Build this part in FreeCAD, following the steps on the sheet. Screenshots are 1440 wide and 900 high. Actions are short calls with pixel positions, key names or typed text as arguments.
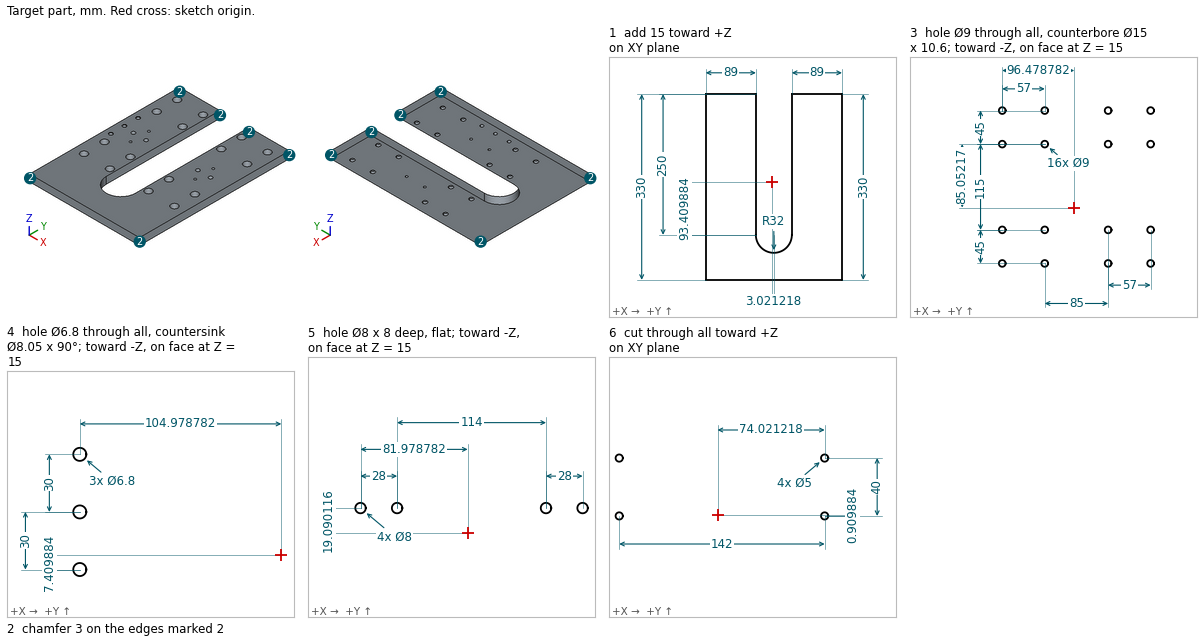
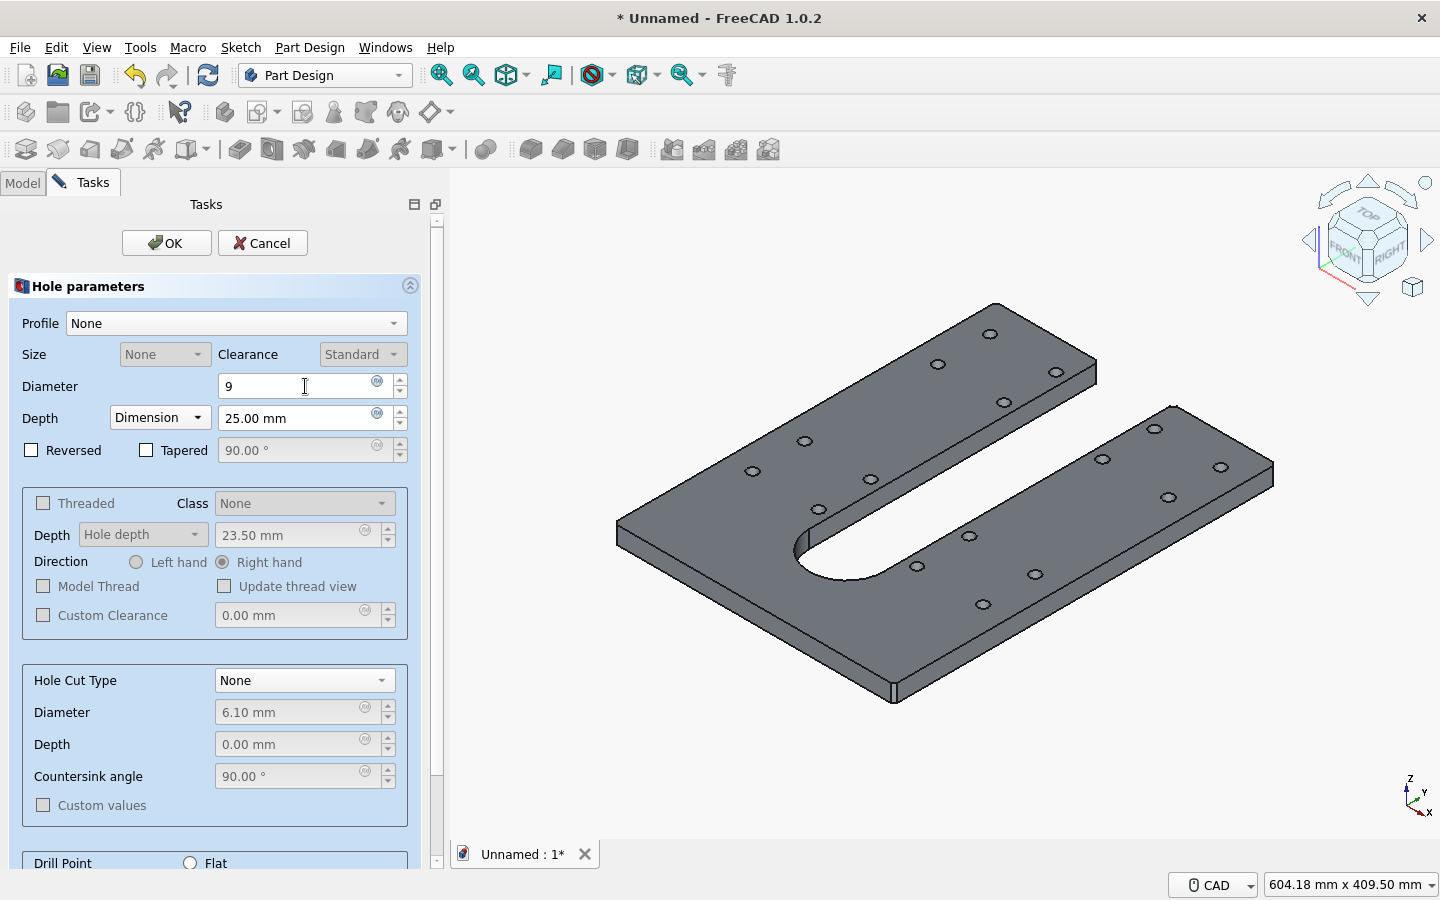
click(161, 418)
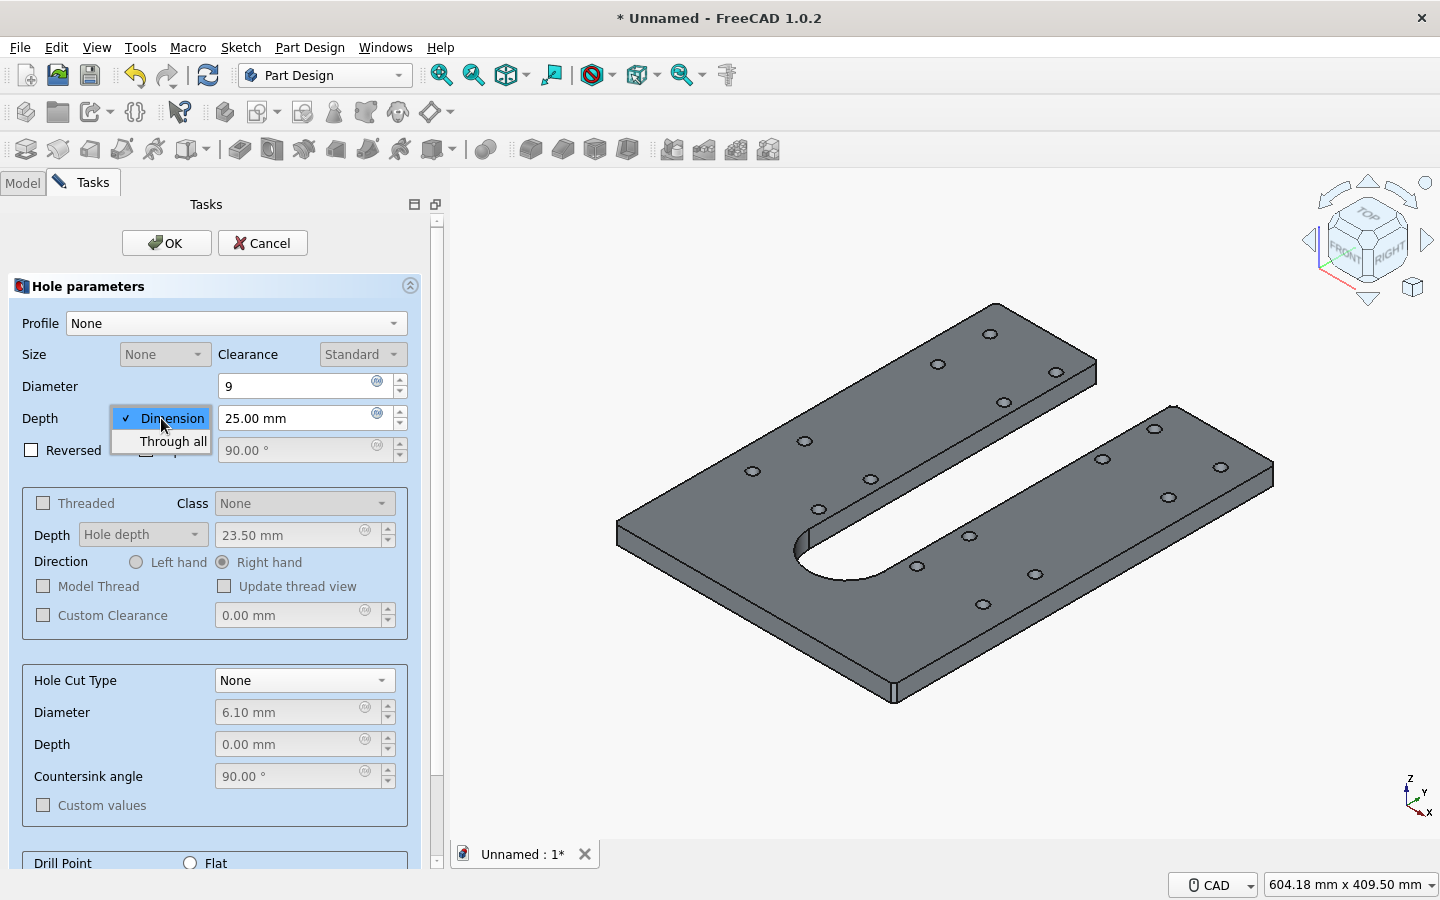
click(160, 442)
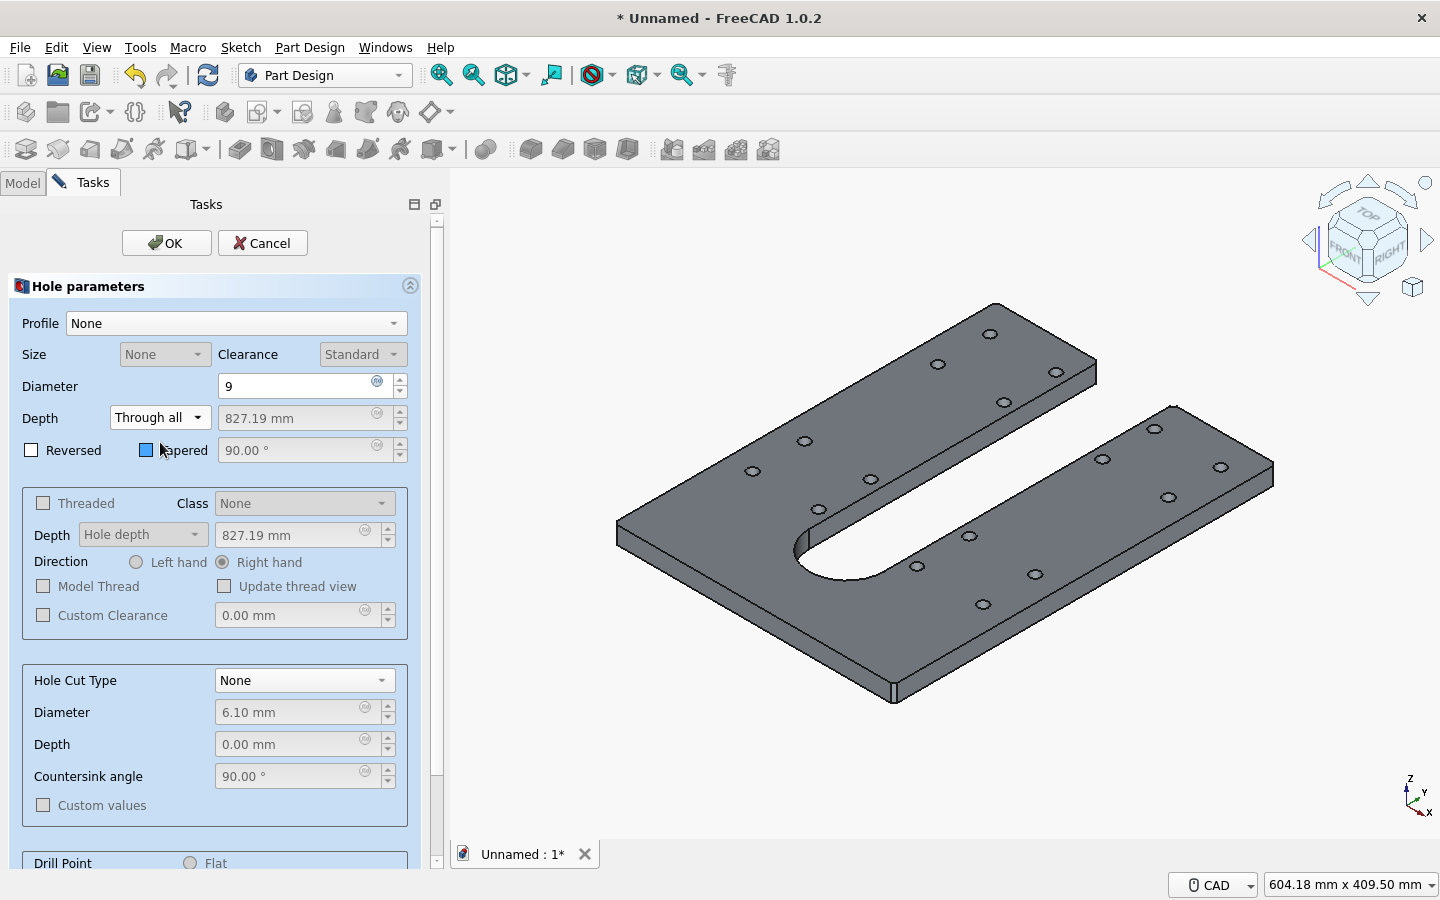
click(306, 680)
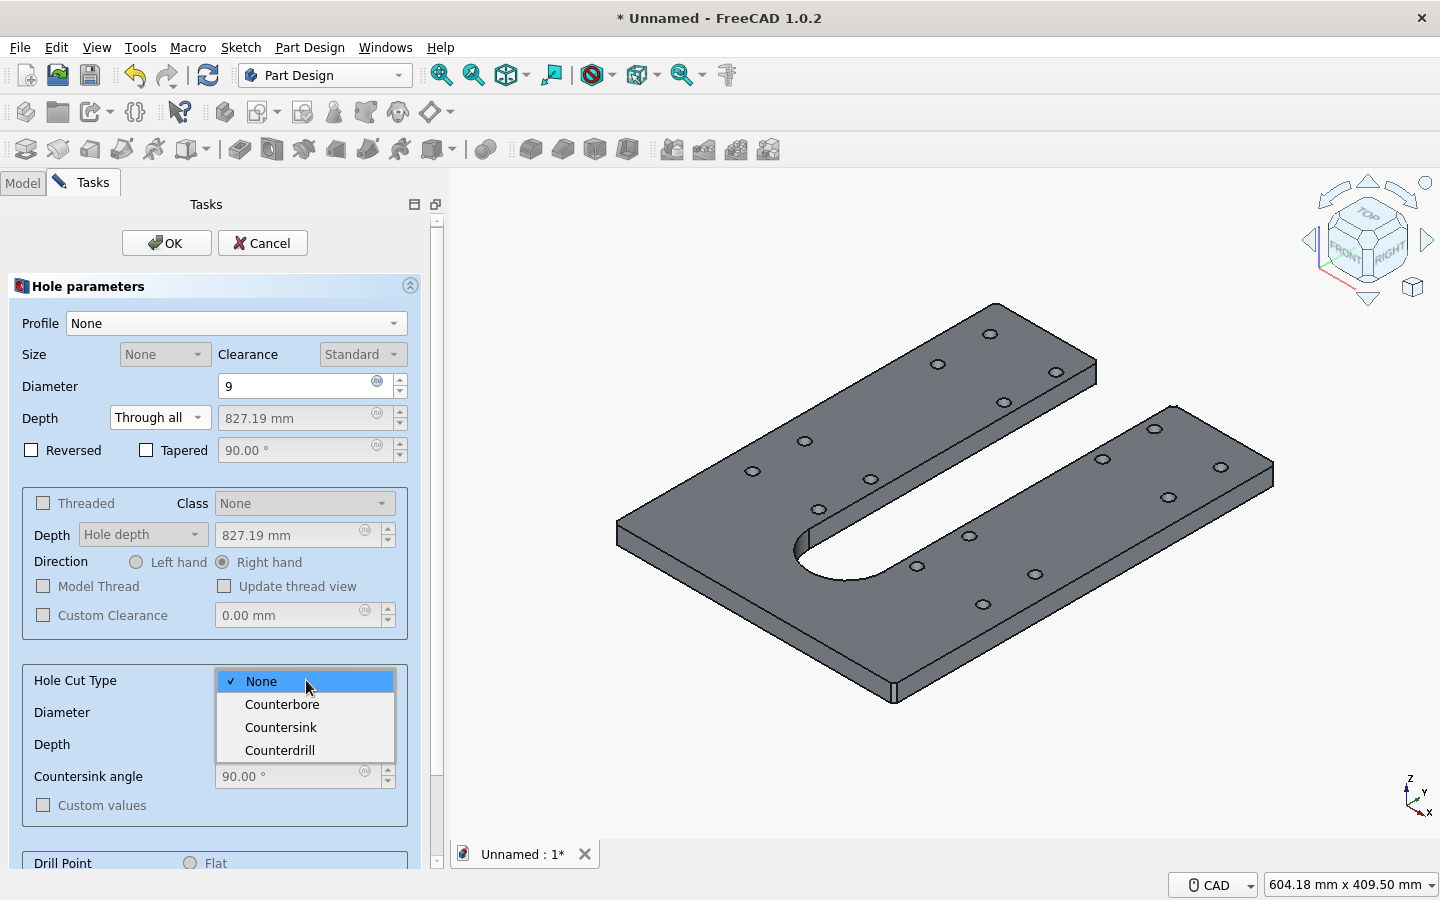
click(304, 704)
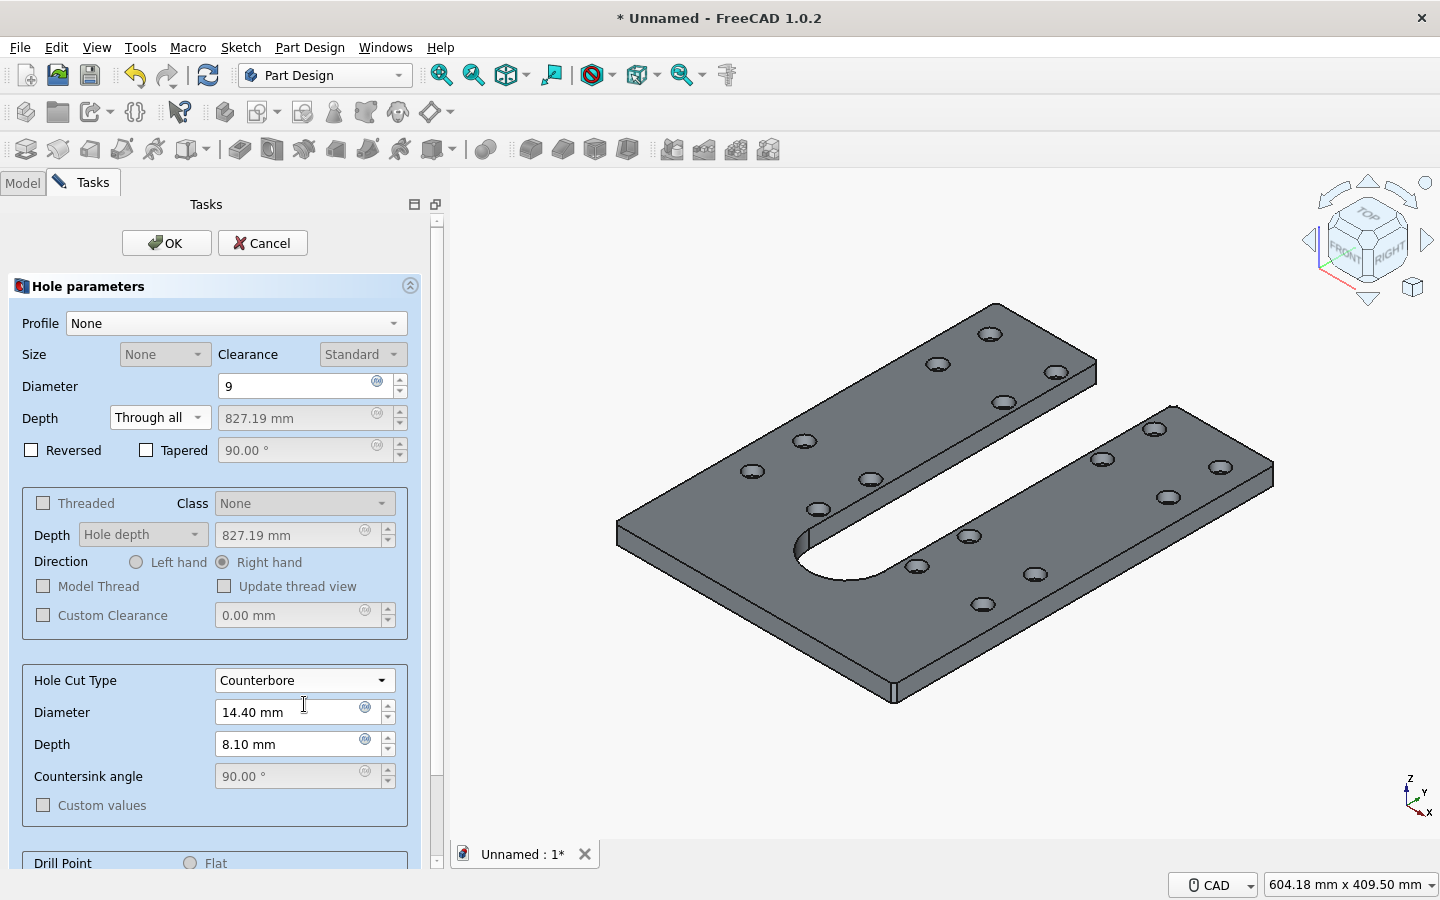
triple_click(298, 712)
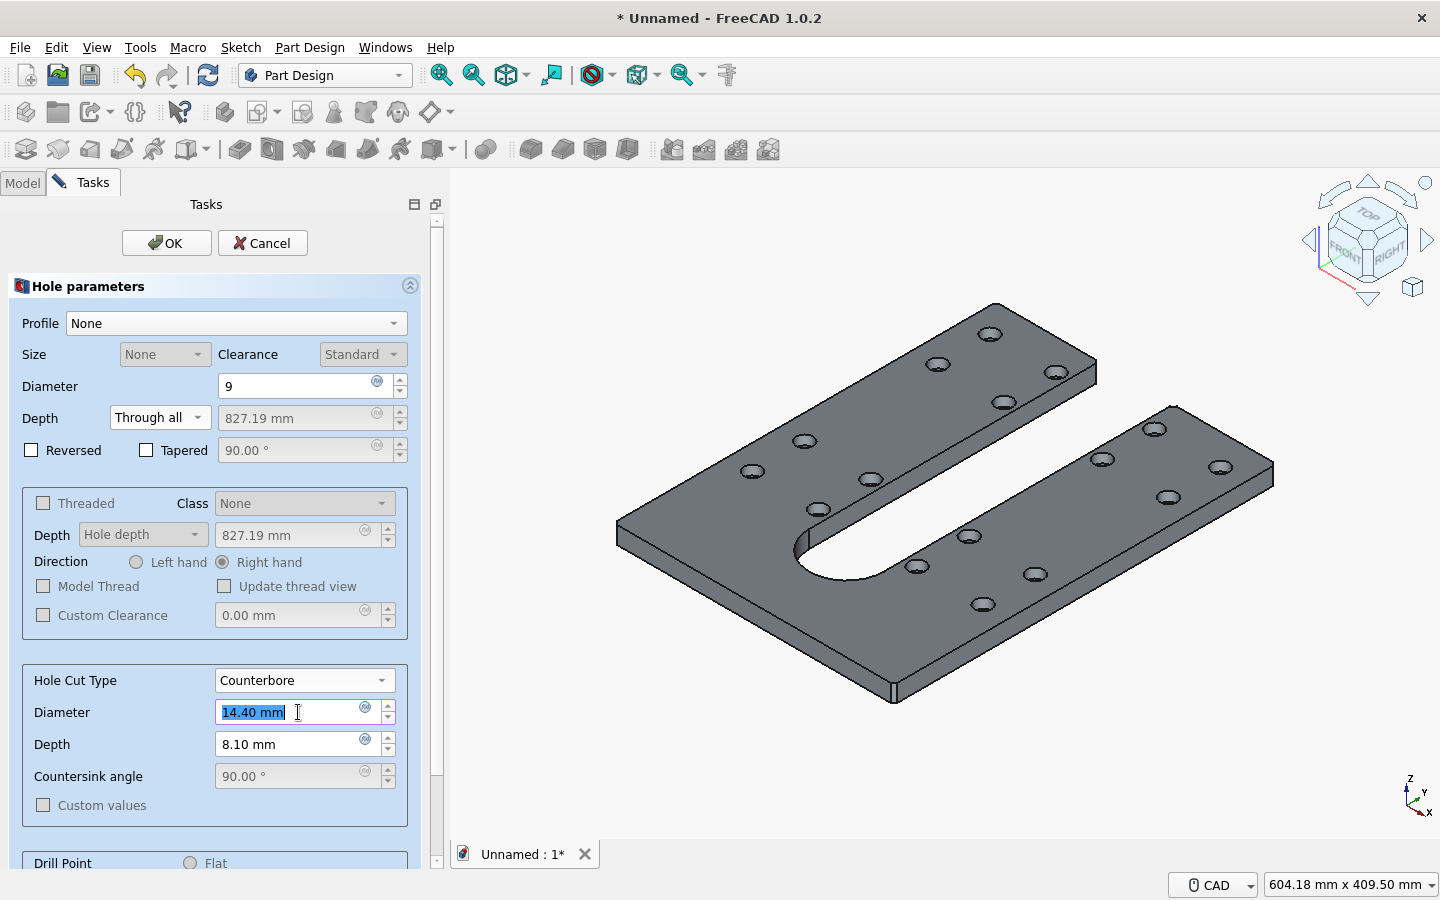
text(15)
key(Tab)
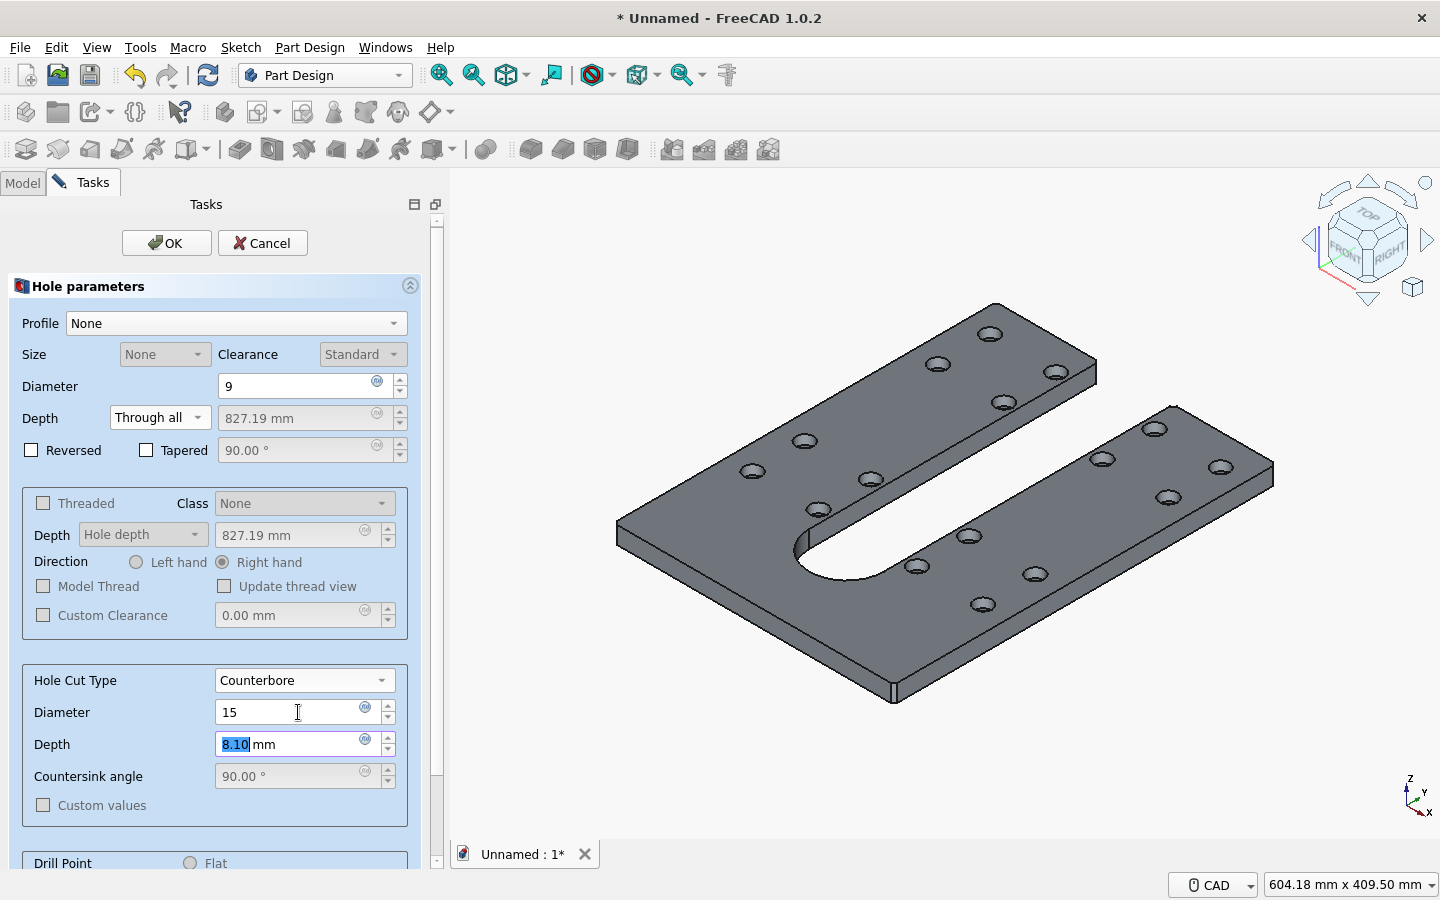
text(10.6)
key(Tab)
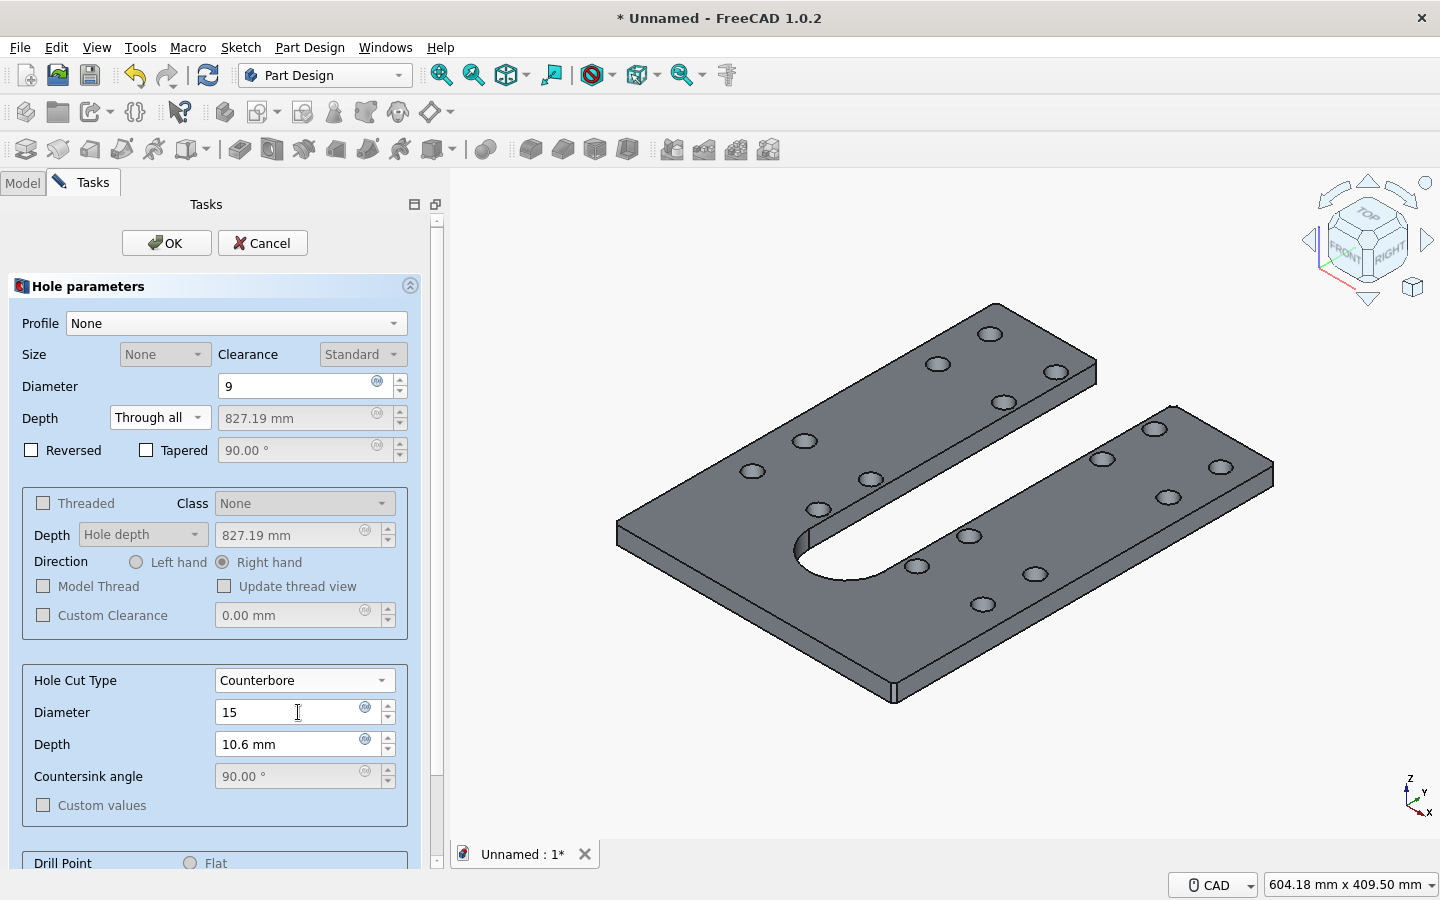
click(167, 243)